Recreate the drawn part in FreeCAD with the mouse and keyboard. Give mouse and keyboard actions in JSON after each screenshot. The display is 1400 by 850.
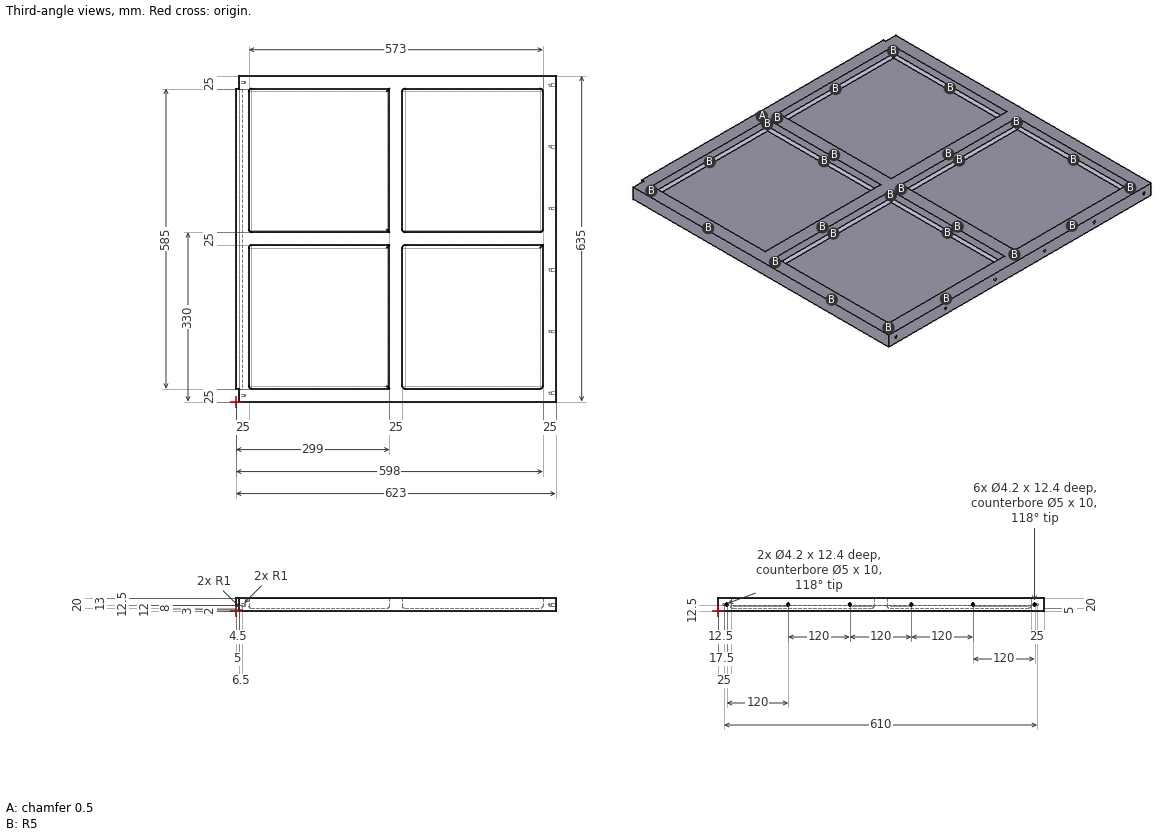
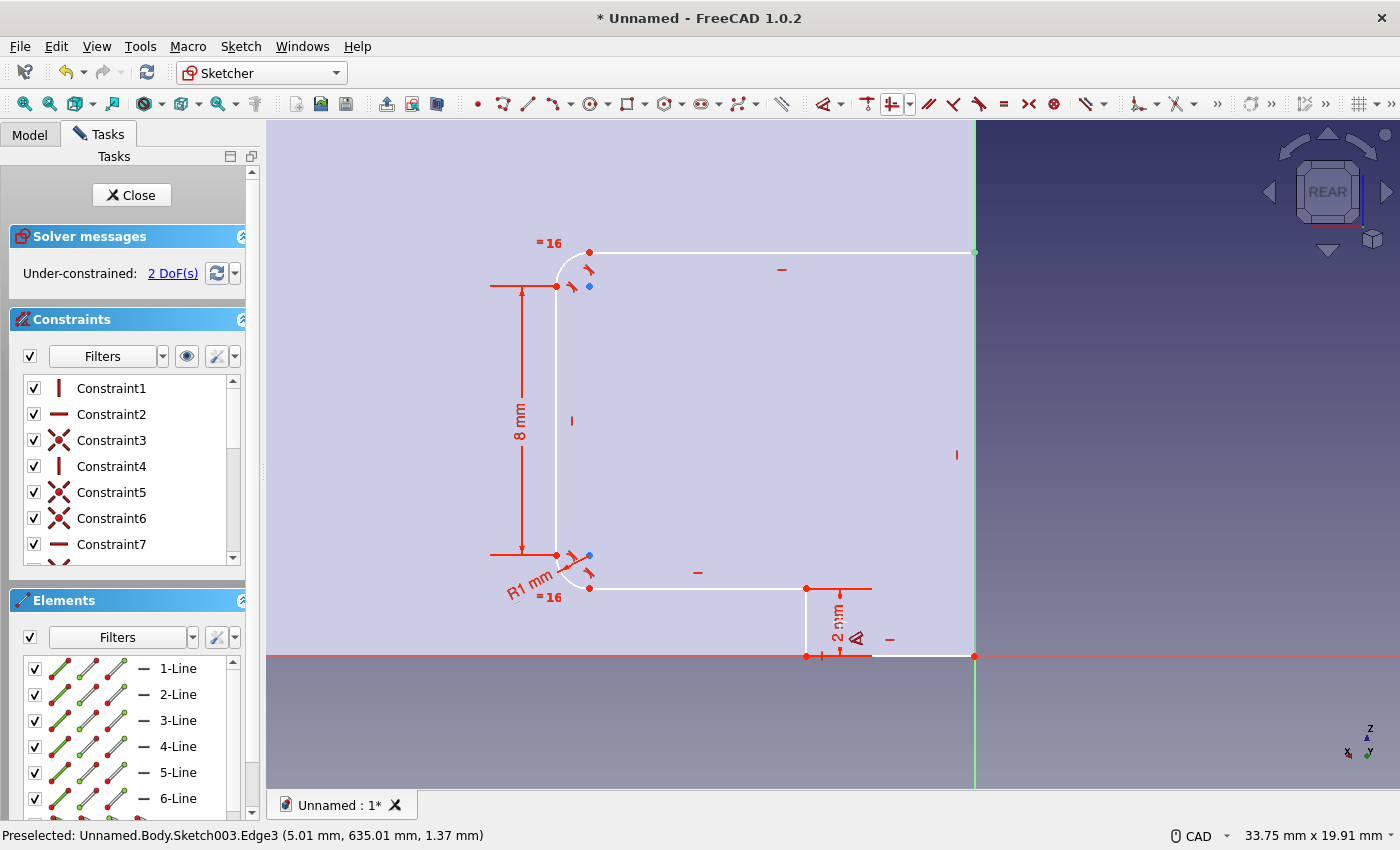
{"action": "left_click", "coordinate": [857, 656]}
{"action": "left_click", "coordinate": [890, 690]}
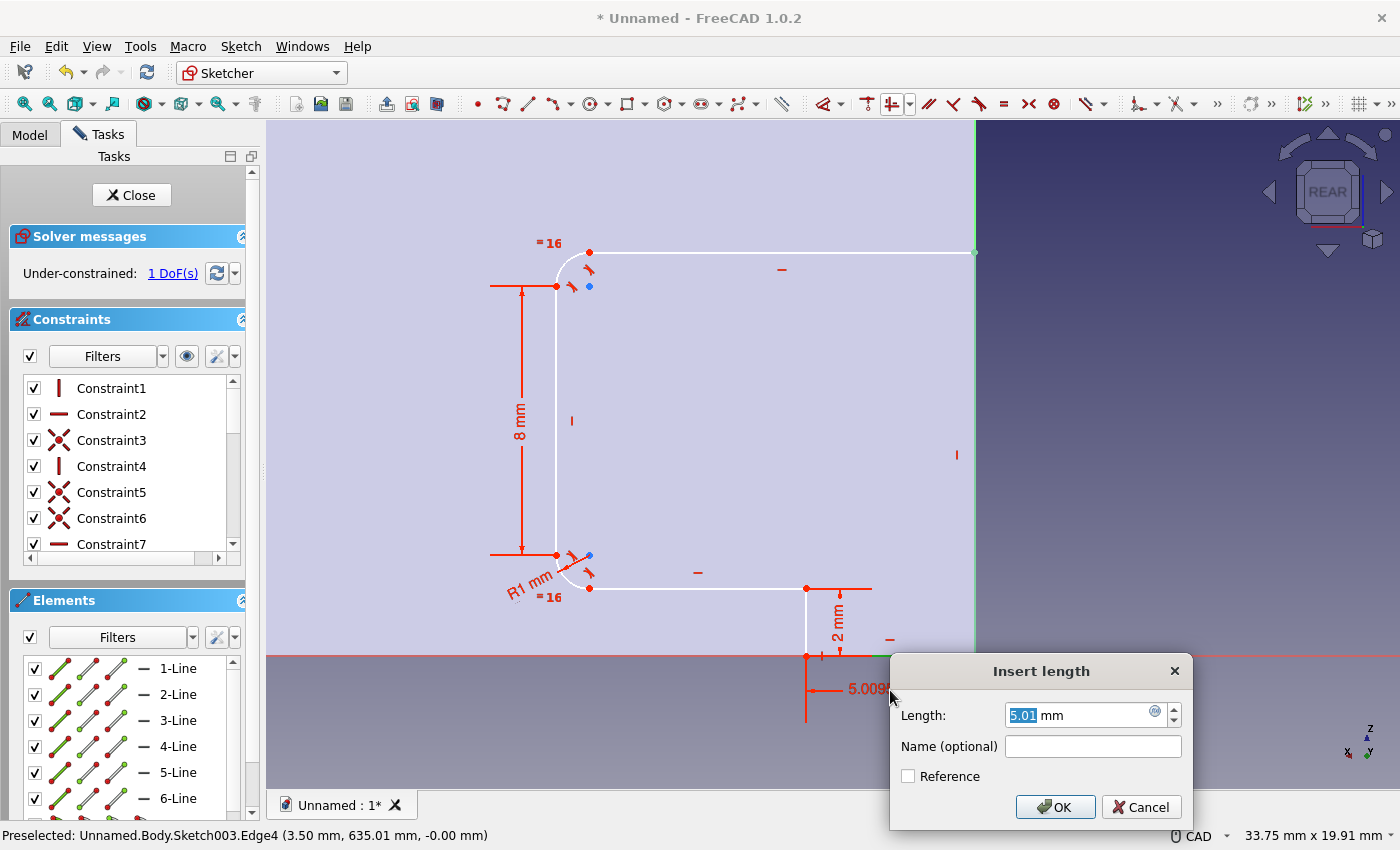
{"action": "type", "text": "5"}
{"action": "key", "text": "Return"}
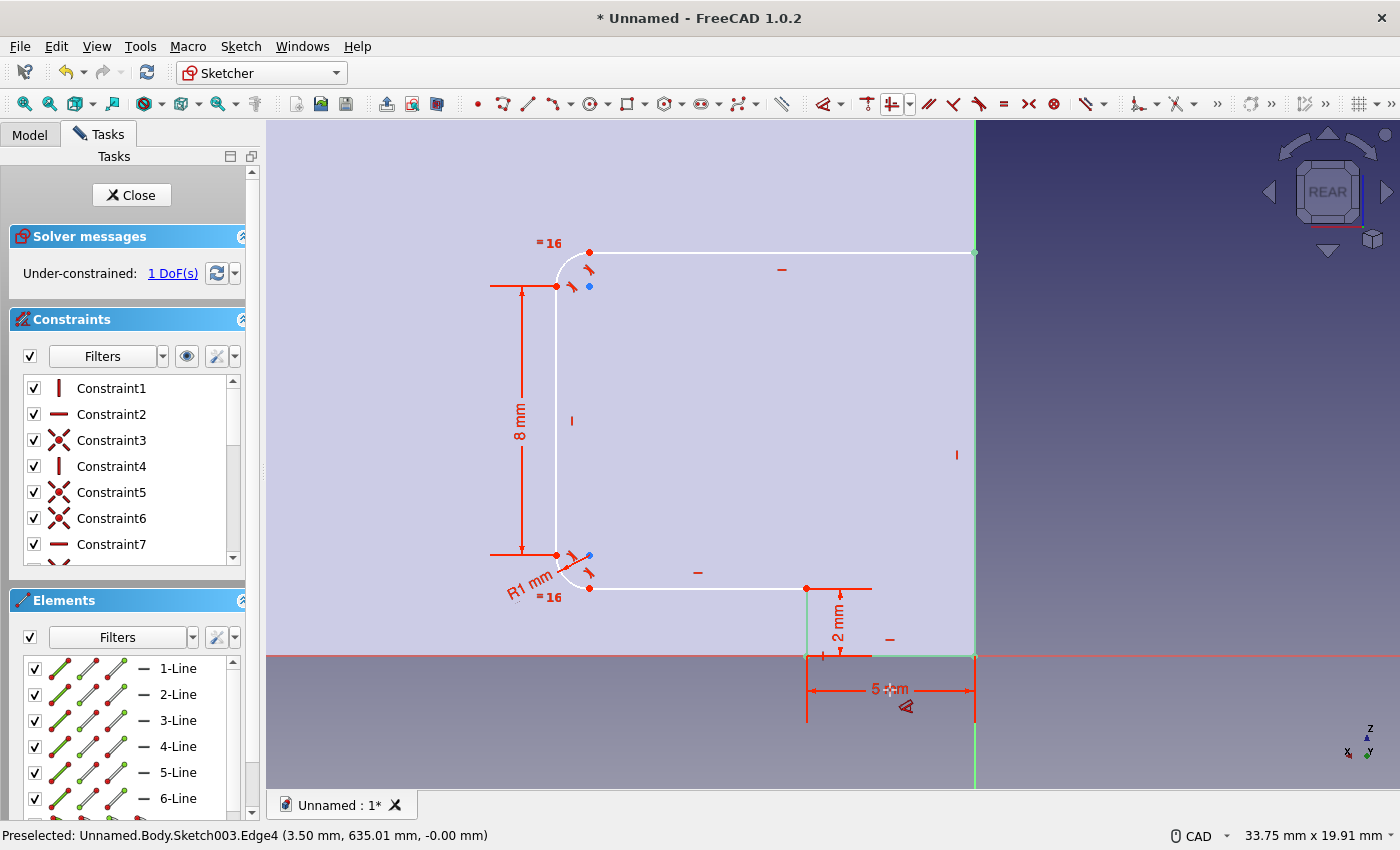
{"action": "left_click", "coordinate": [655, 589]}
{"action": "left_click", "coordinate": [698, 623]}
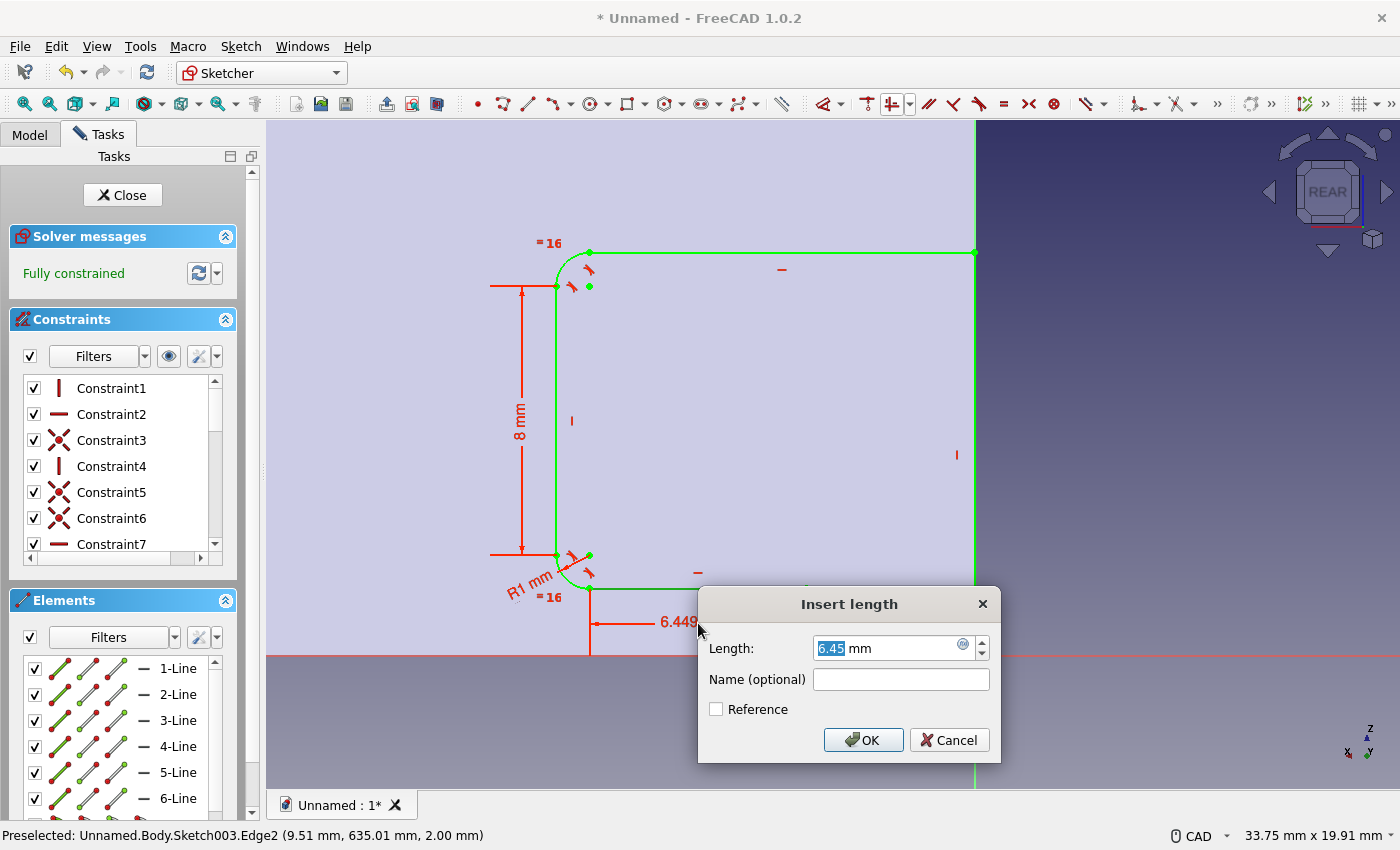
{"action": "type", "text": "6.5"}
{"action": "key", "text": "Return"}
{"action": "key", "text": "Escape"}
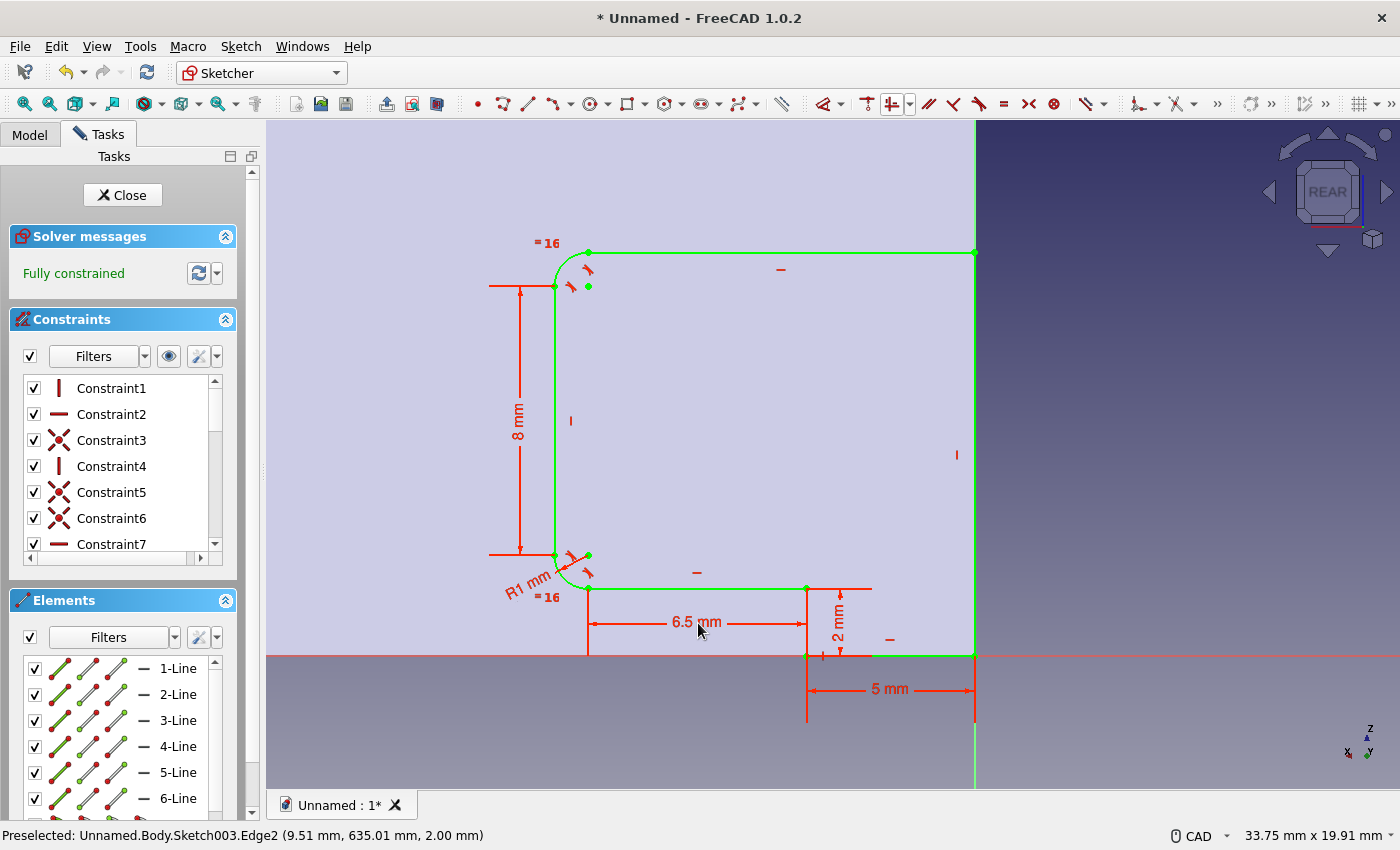
{"action": "left_click", "coordinate": [123, 195]}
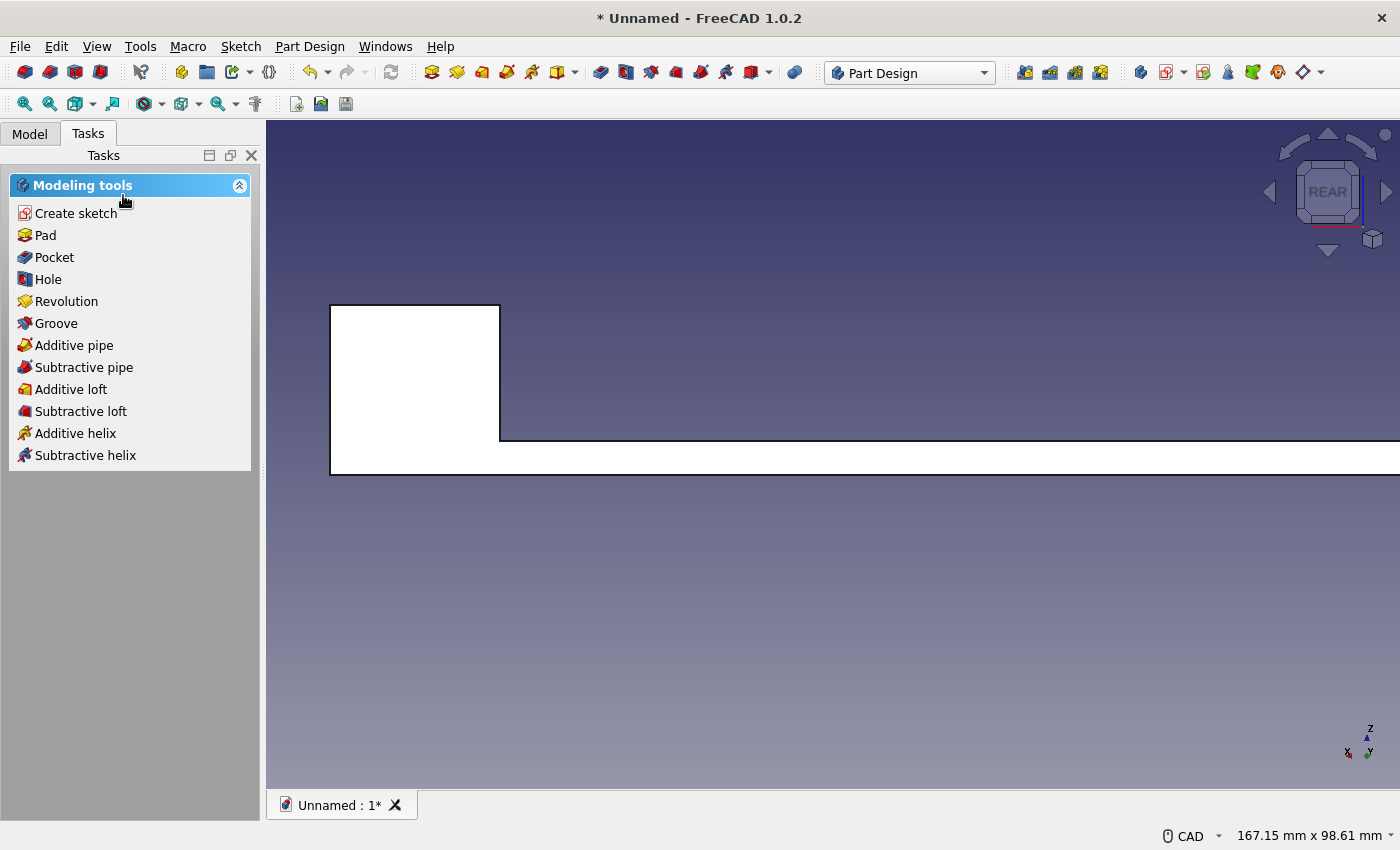
{"action": "left_click", "coordinate": [601, 72]}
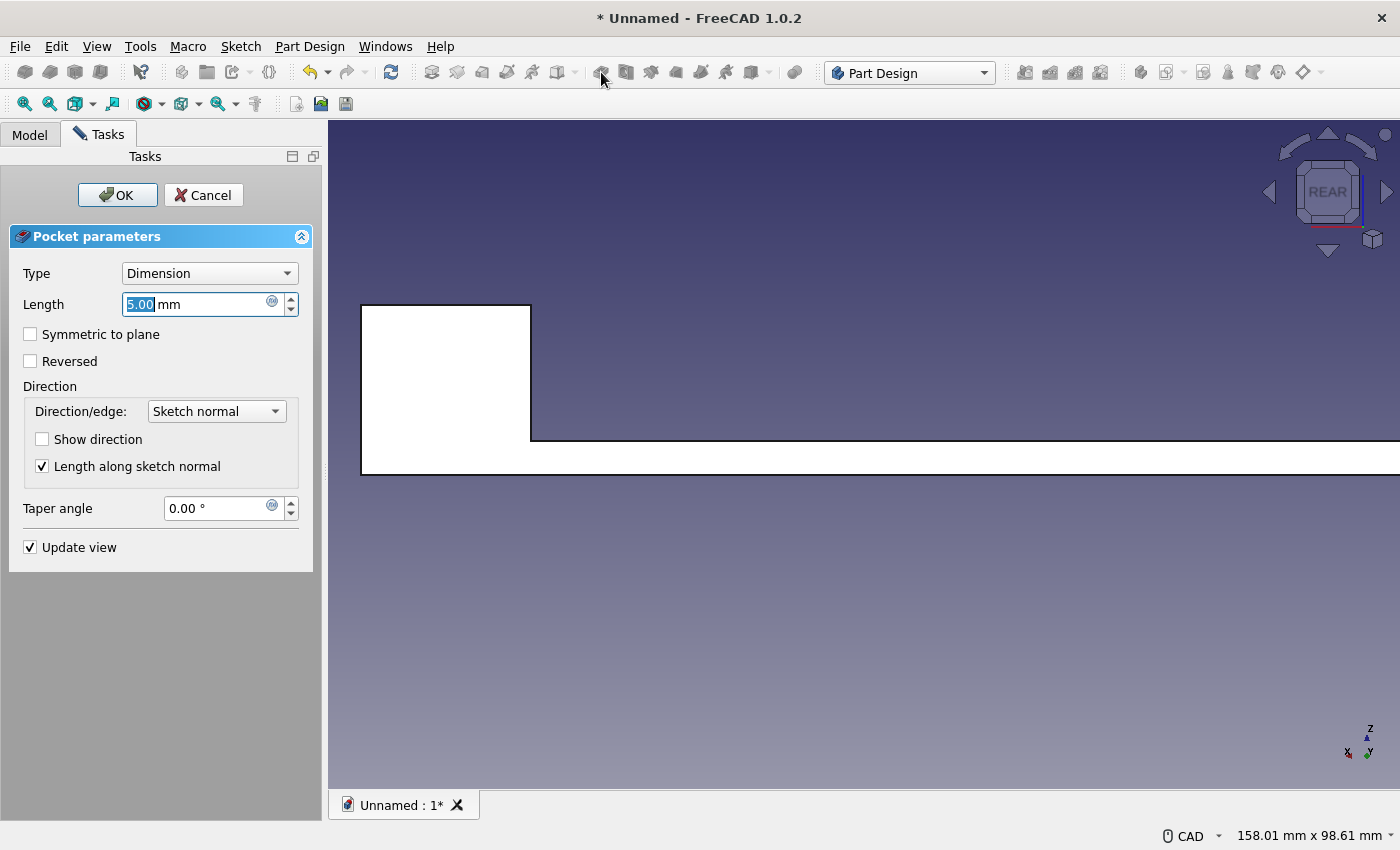
{"action": "left_click", "coordinate": [210, 274]}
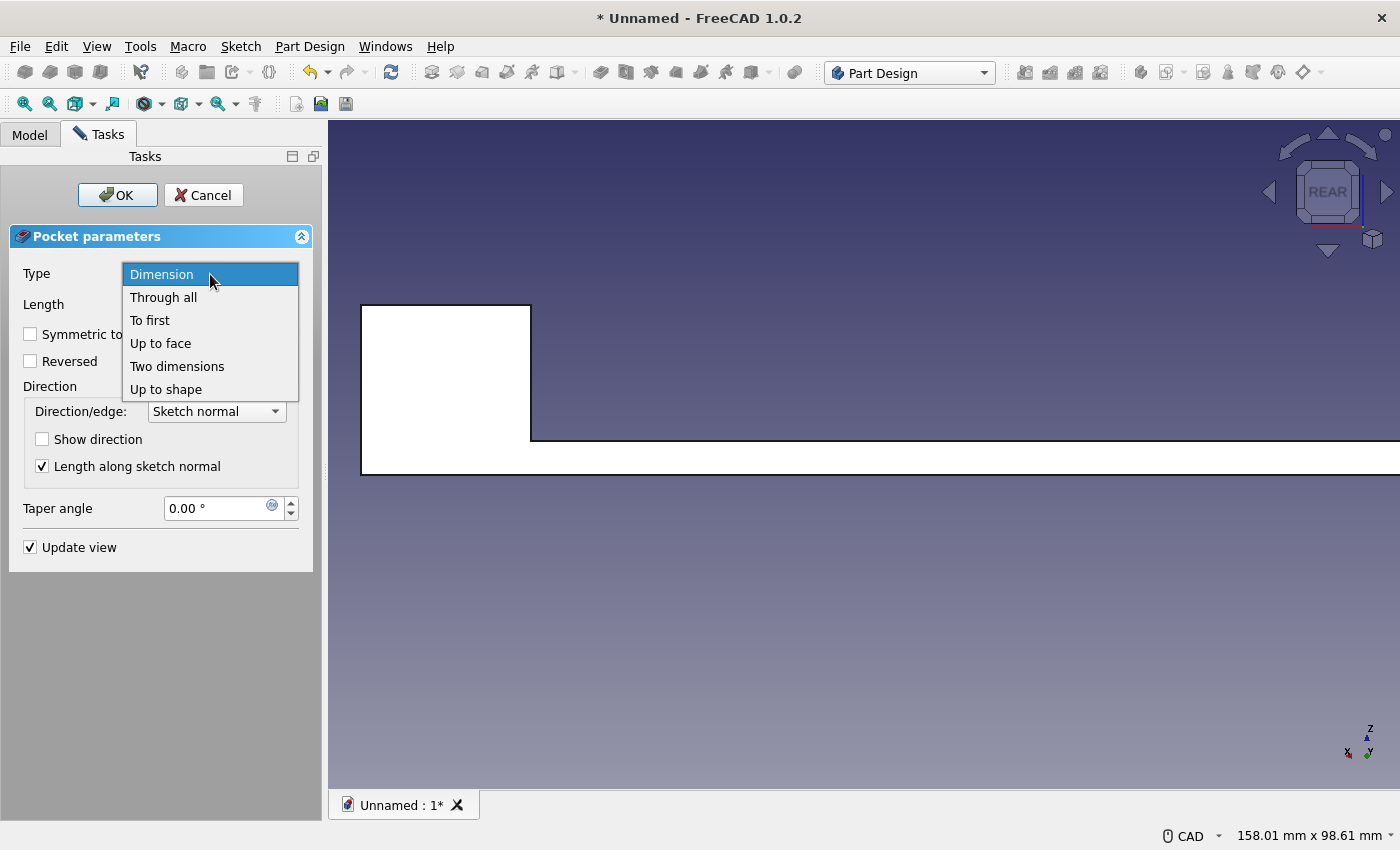
{"action": "left_click", "coordinate": [208, 298]}